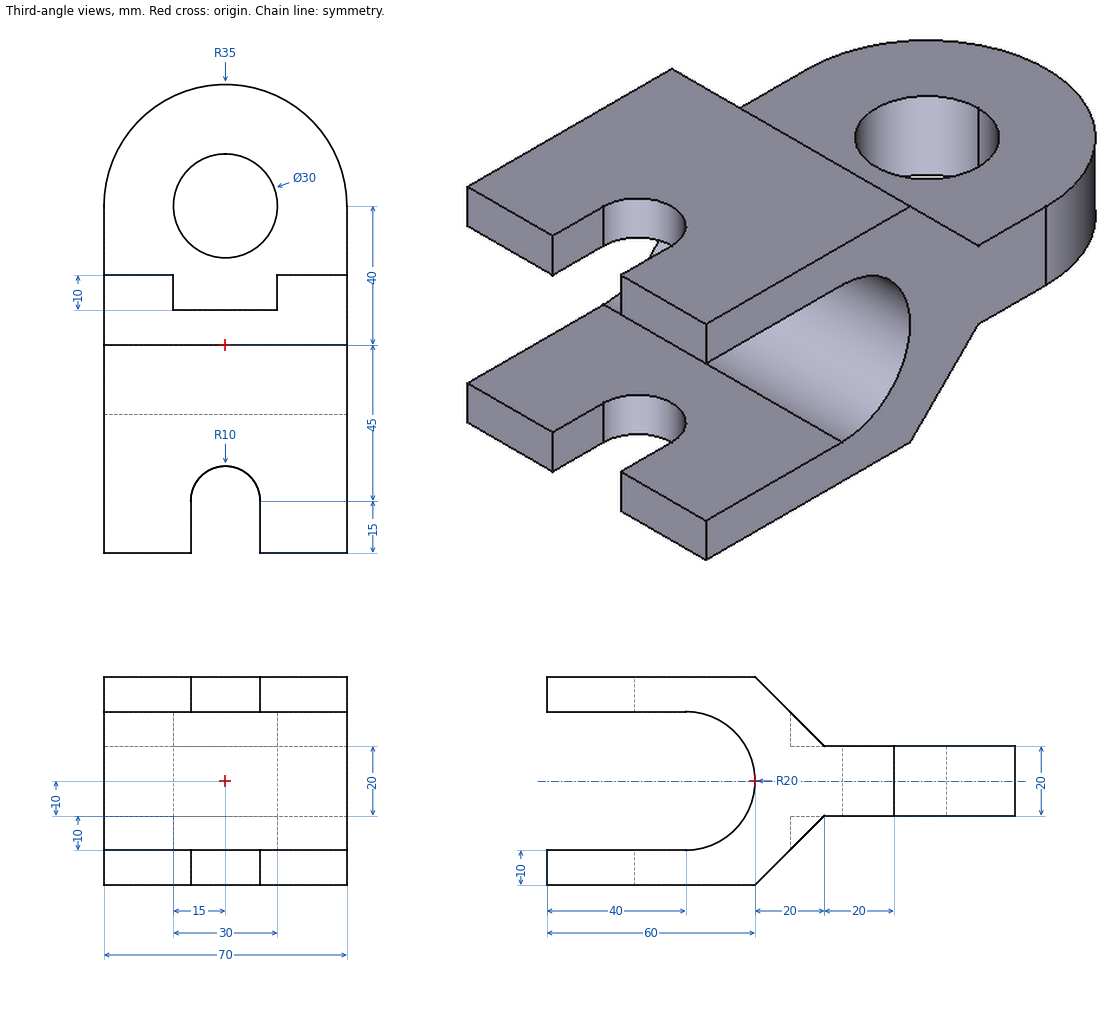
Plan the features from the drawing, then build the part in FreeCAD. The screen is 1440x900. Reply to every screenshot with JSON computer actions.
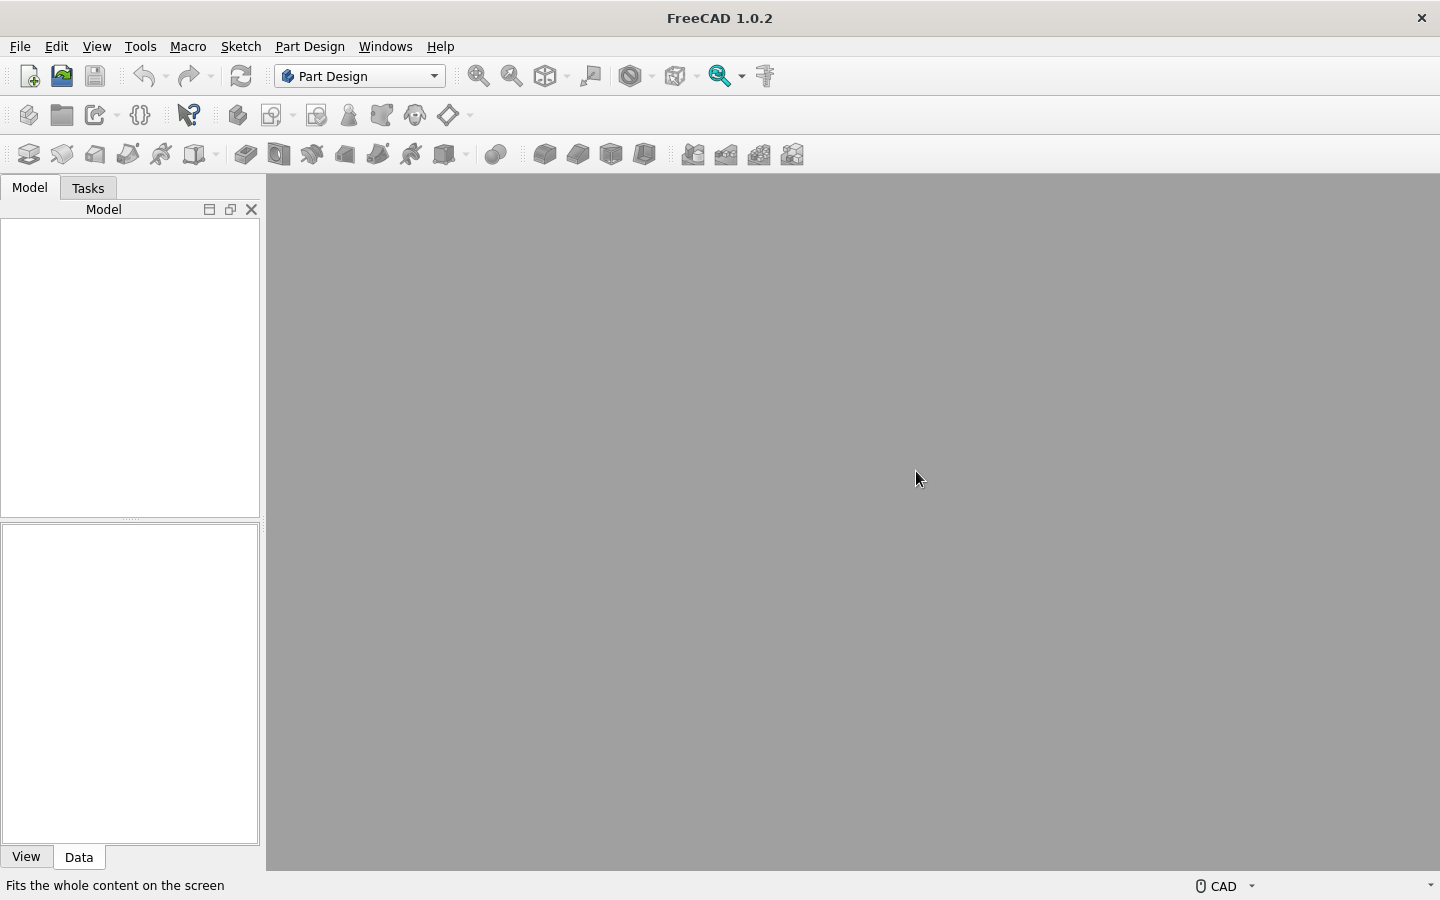
{"action": "key", "text": "ctrl+n"}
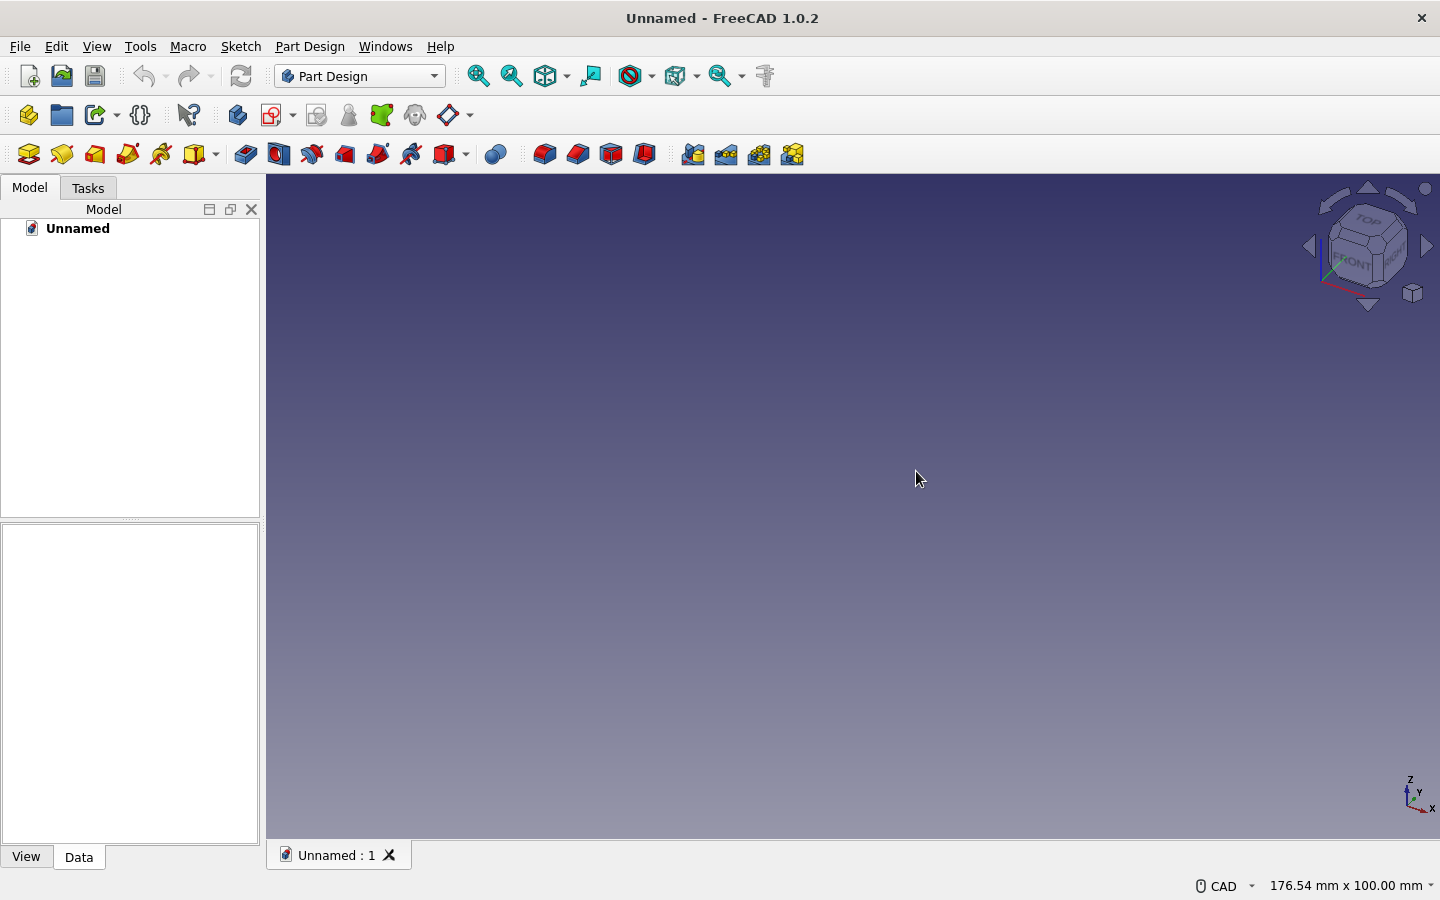
{"action": "left_click", "coordinate": [270, 116]}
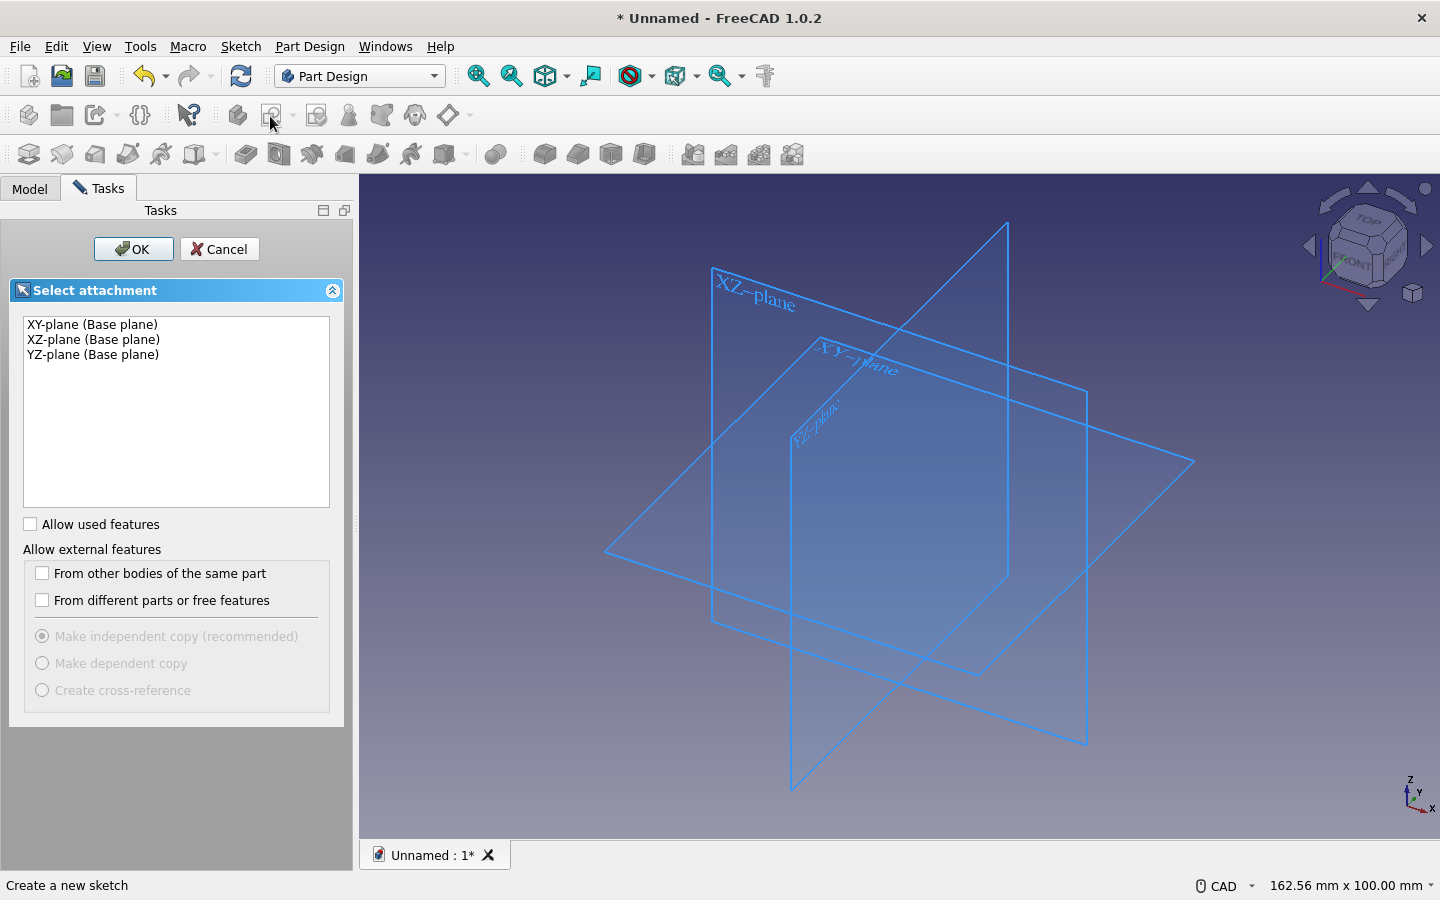
{"action": "left_click", "coordinate": [84, 354]}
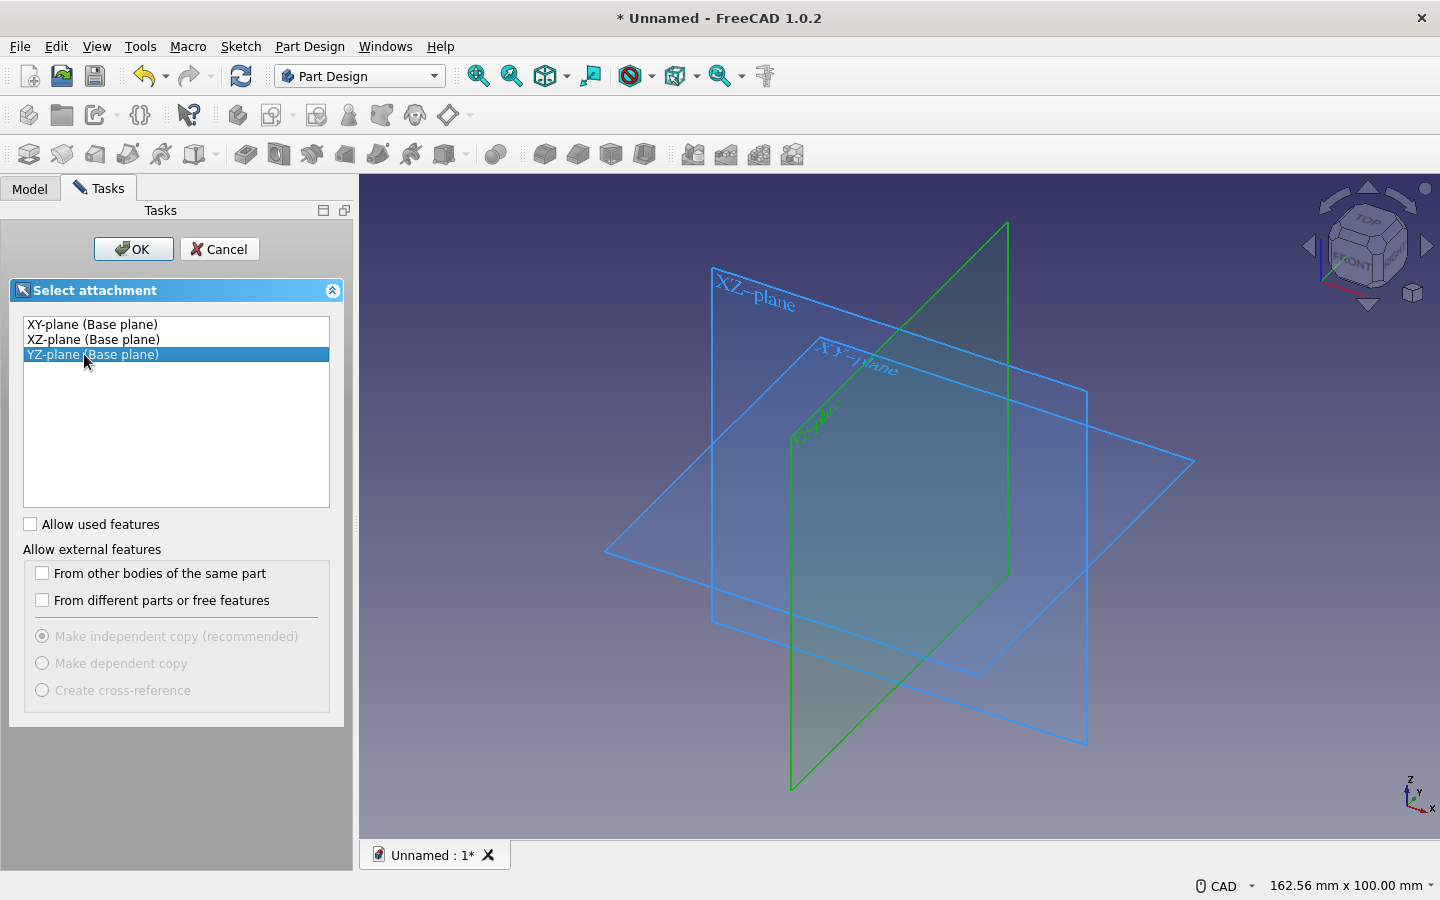
{"action": "left_click", "coordinate": [134, 249]}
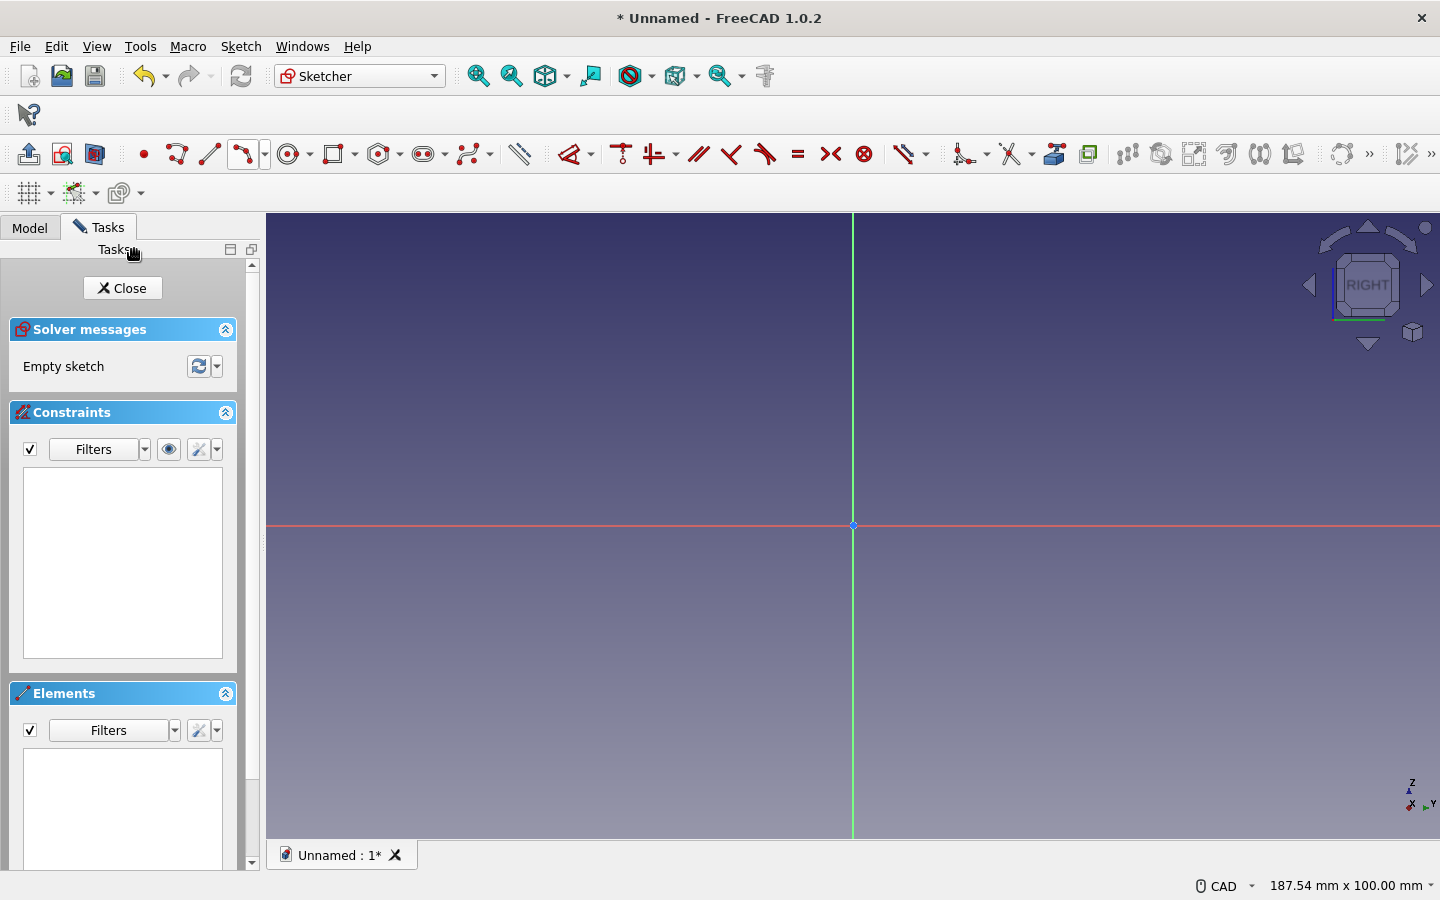
{"action": "key", "text": "g m"}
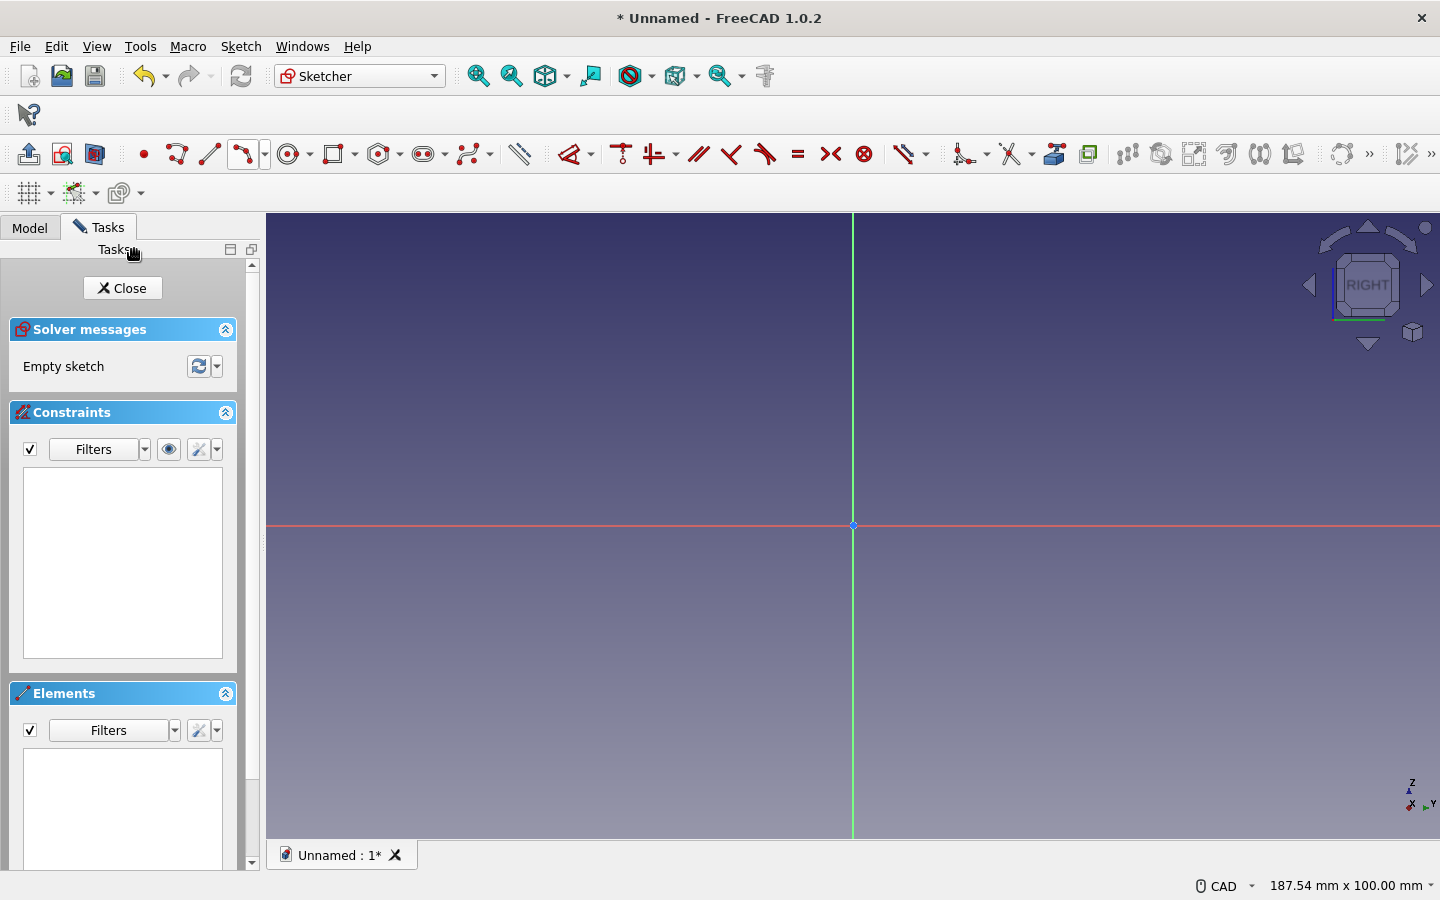
{"action": "left_click", "coordinate": [728, 651]}
{"action": "left_click", "coordinate": [477, 651]}
{"action": "left_click", "coordinate": [477, 714]}
{"action": "left_click", "coordinate": [853, 714]}
{"action": "left_click", "coordinate": [978, 589]}
{"action": "left_click", "coordinate": [1103, 589]}
{"action": "left_click", "coordinate": [1103, 463]}
{"action": "left_click", "coordinate": [978, 463]}
{"action": "left_click", "coordinate": [853, 338]}
{"action": "left_click", "coordinate": [477, 338]}
{"action": "left_click", "coordinate": [477, 401]}
{"action": "left_click", "coordinate": [728, 401]}
{"action": "right_click", "coordinate": [728, 401]}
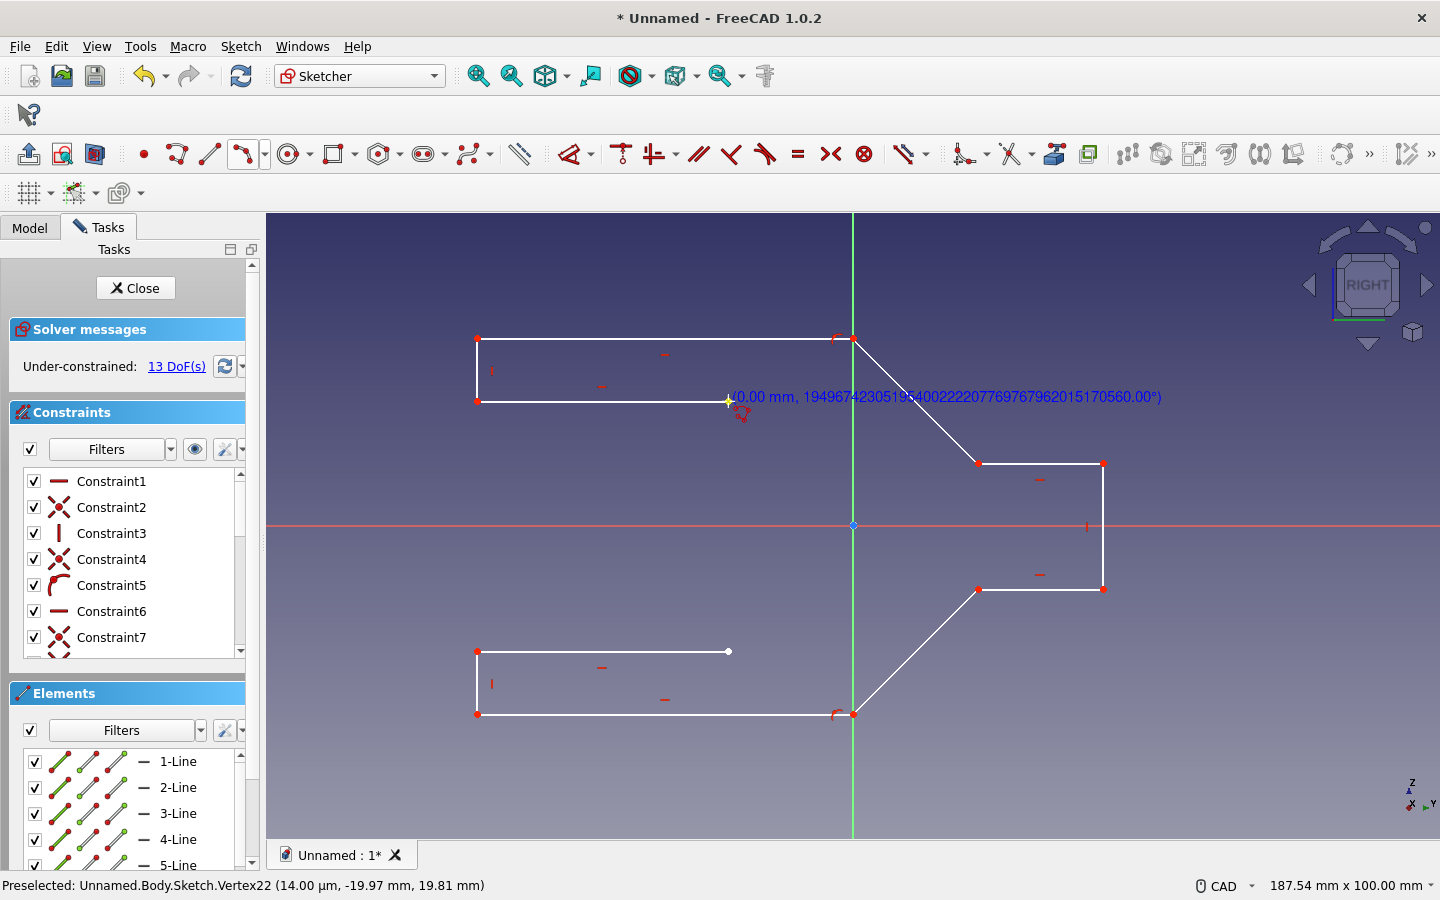
{"action": "key", "text": "g 3 a"}